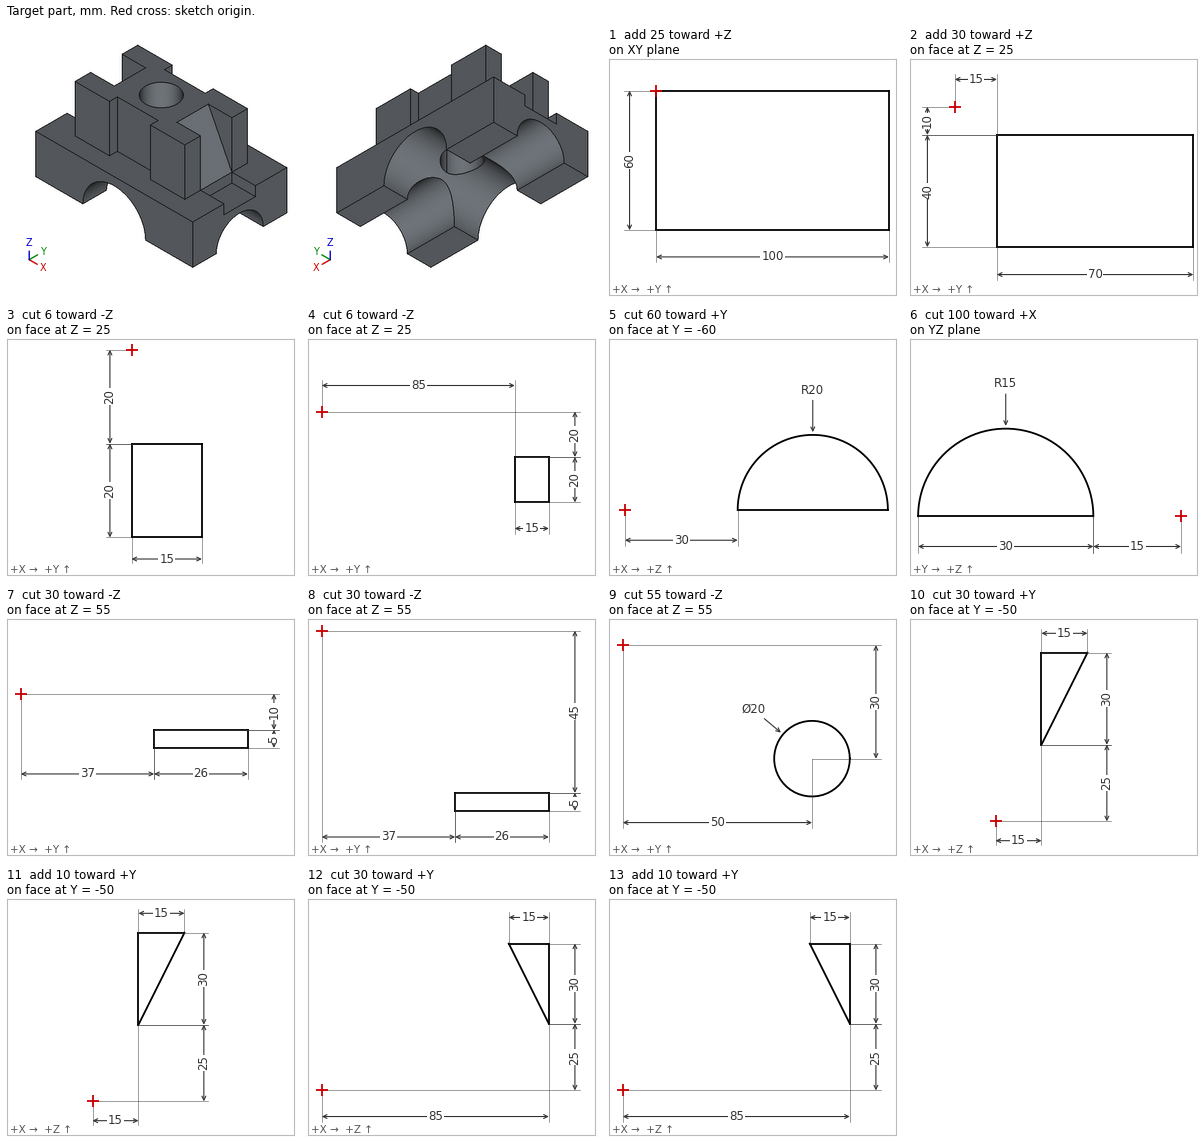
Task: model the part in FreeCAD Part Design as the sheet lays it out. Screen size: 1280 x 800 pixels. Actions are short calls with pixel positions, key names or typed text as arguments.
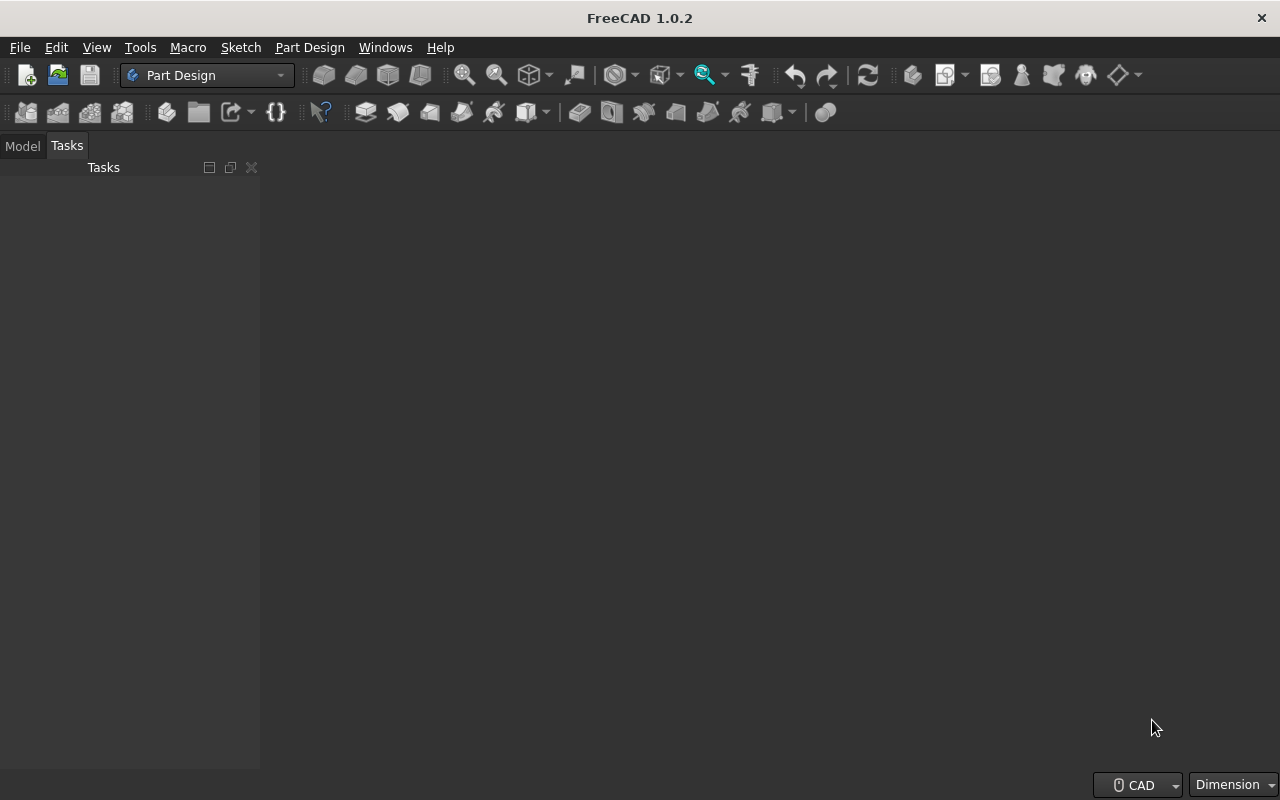
key(ctrl+n)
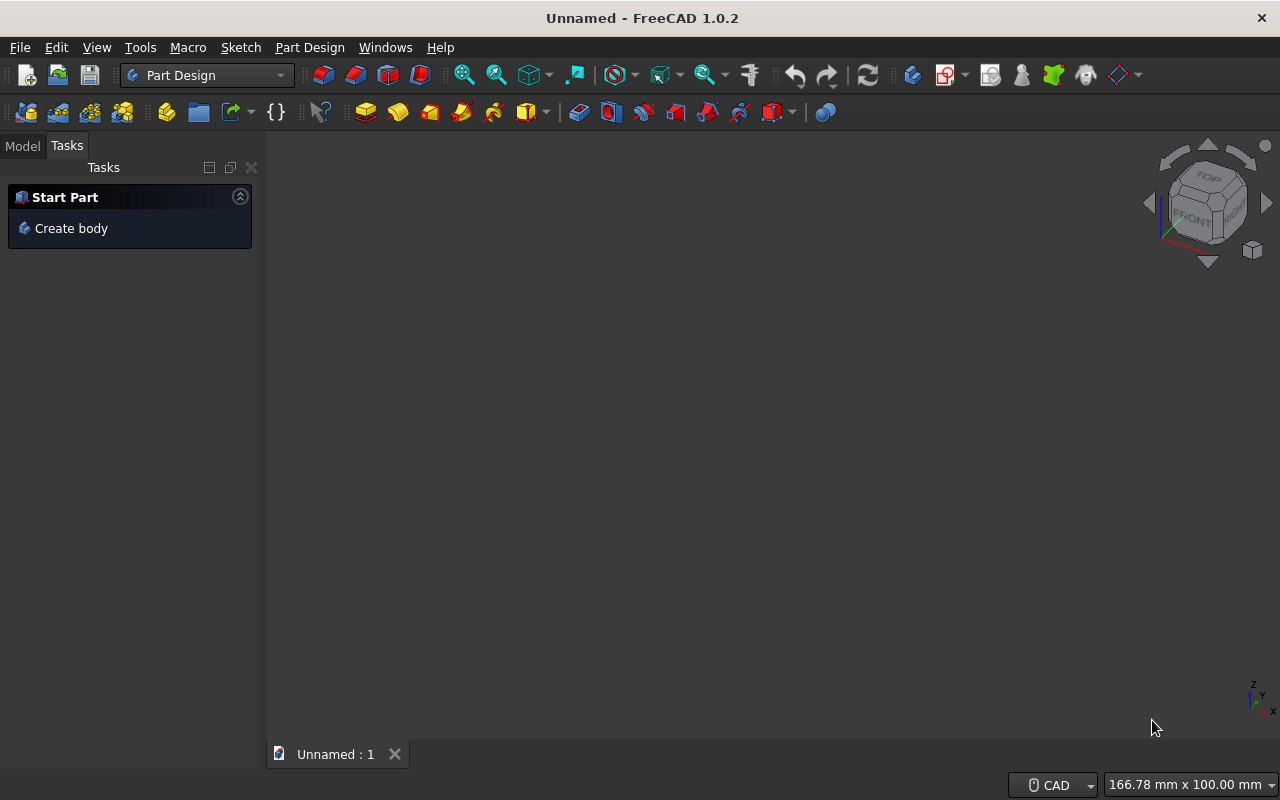
click(946, 76)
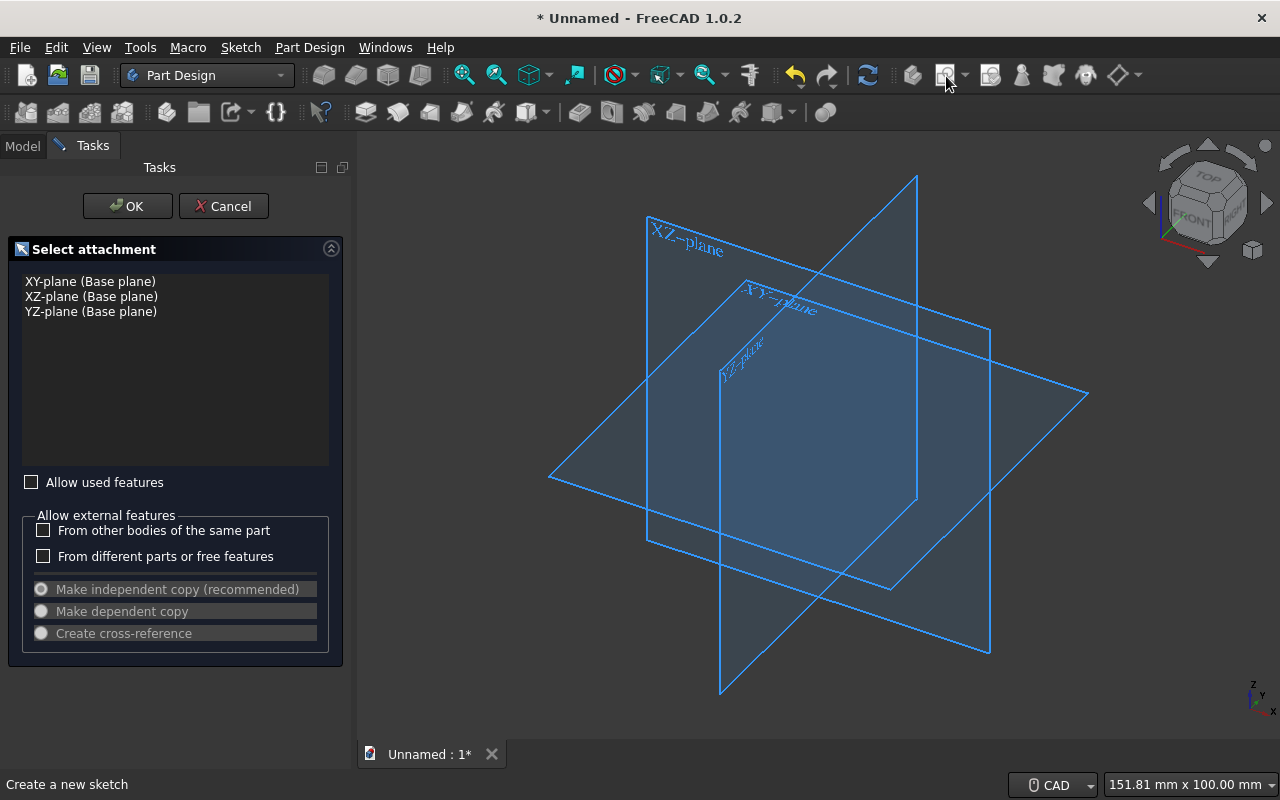
click(82, 282)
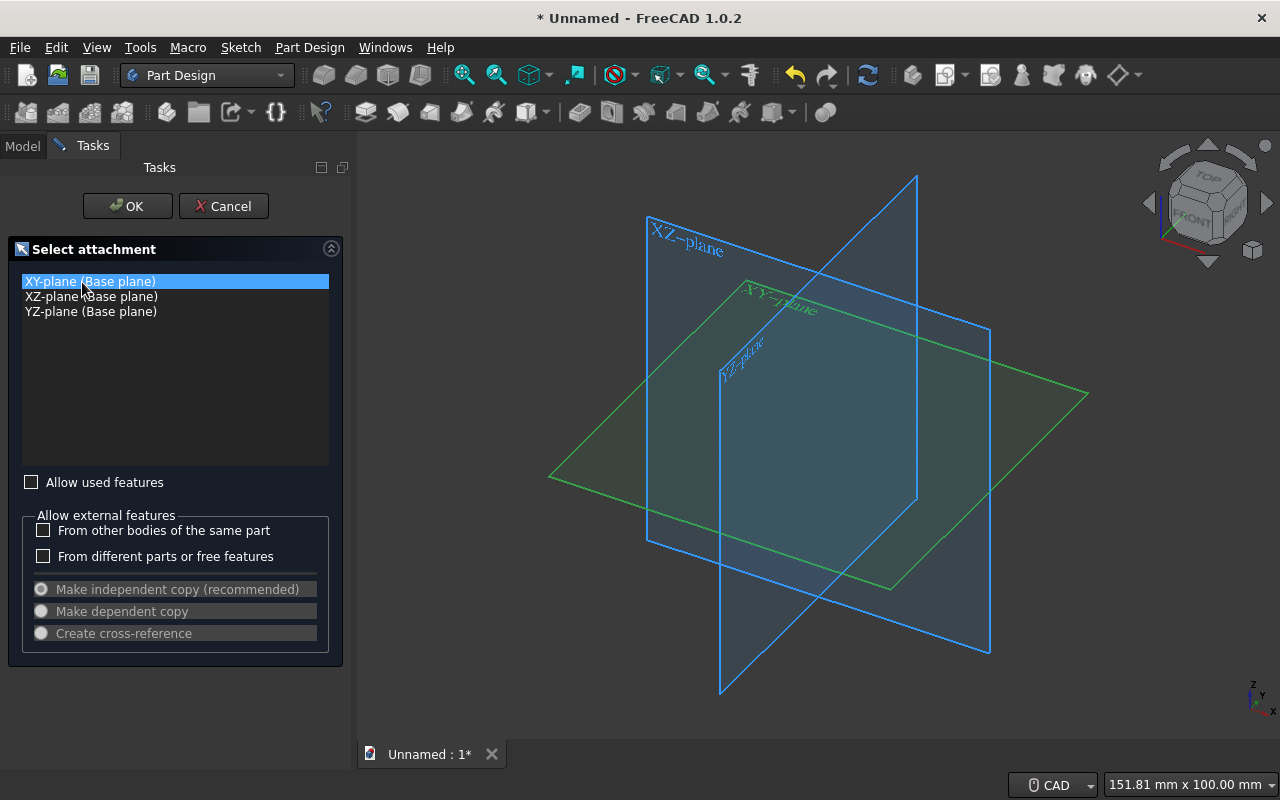
click(128, 206)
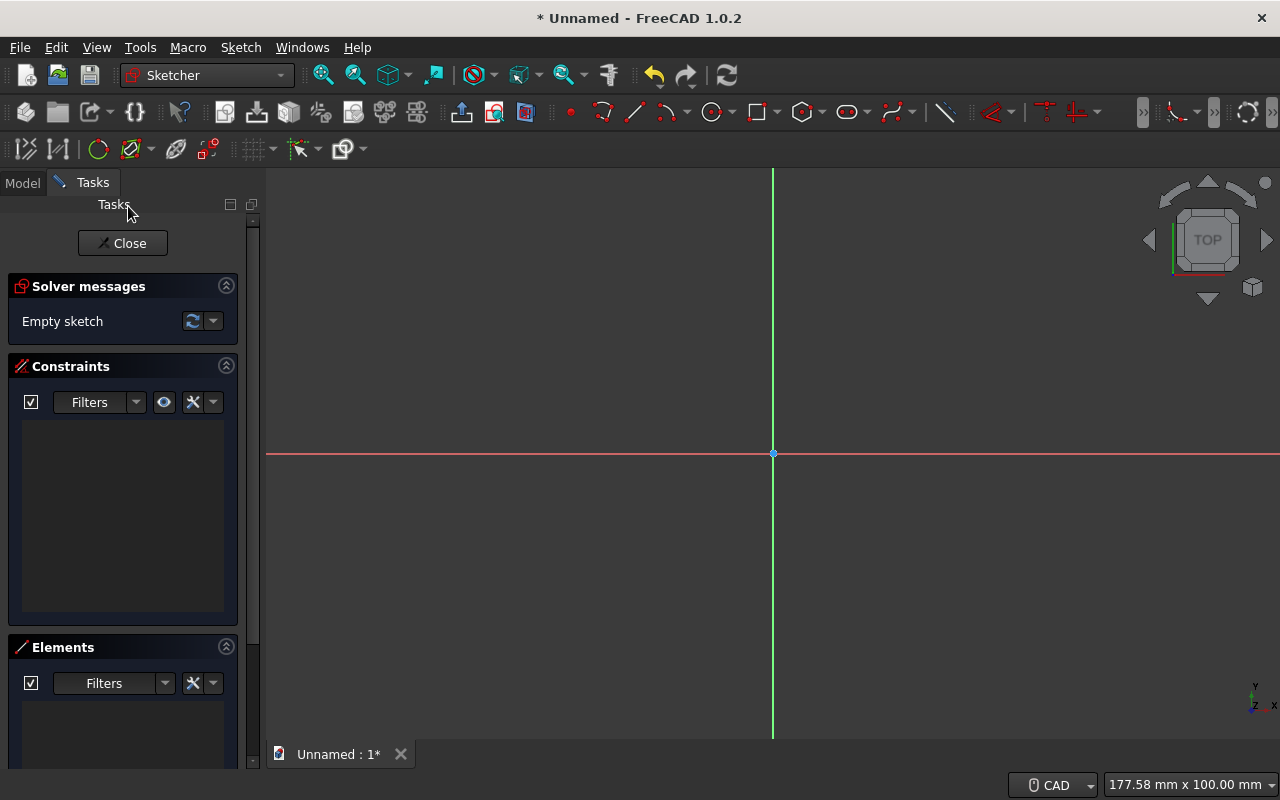
scroll(294, 196, down, 2)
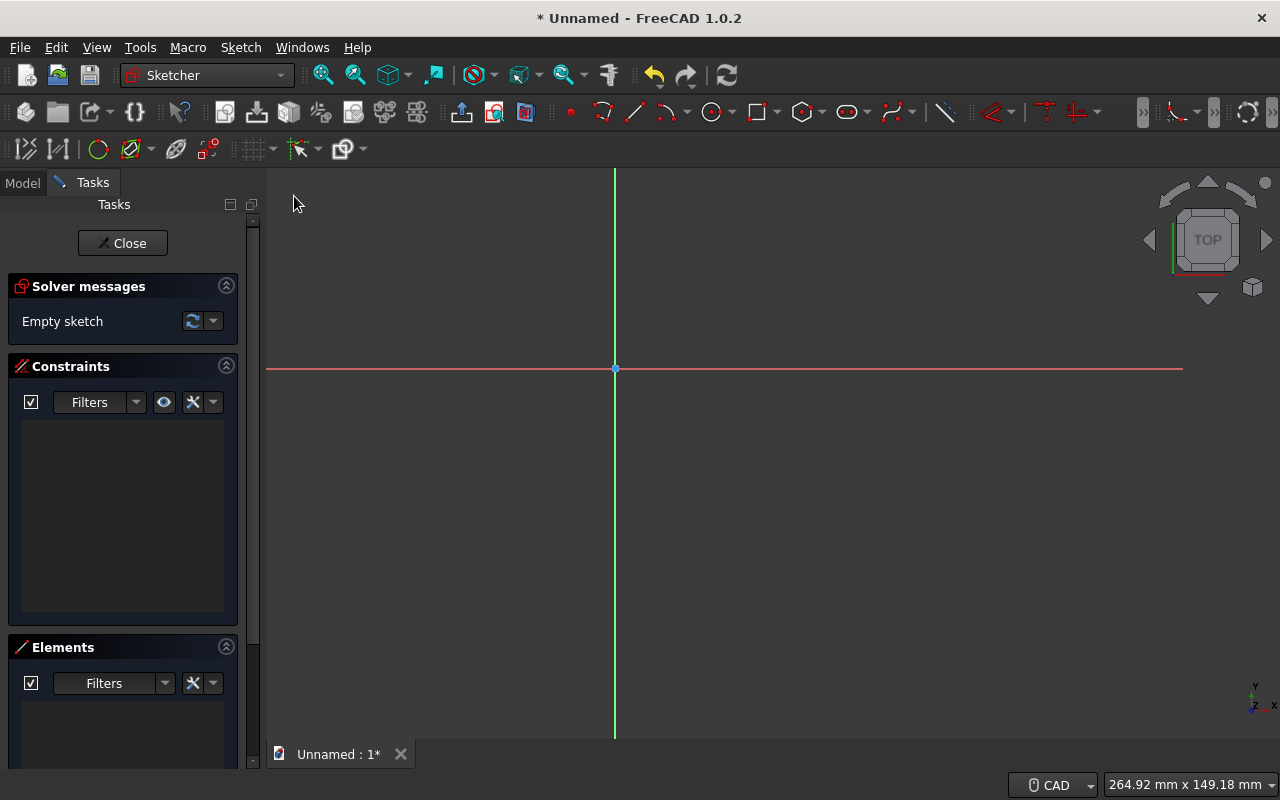
scroll(1014, 544, up, 2)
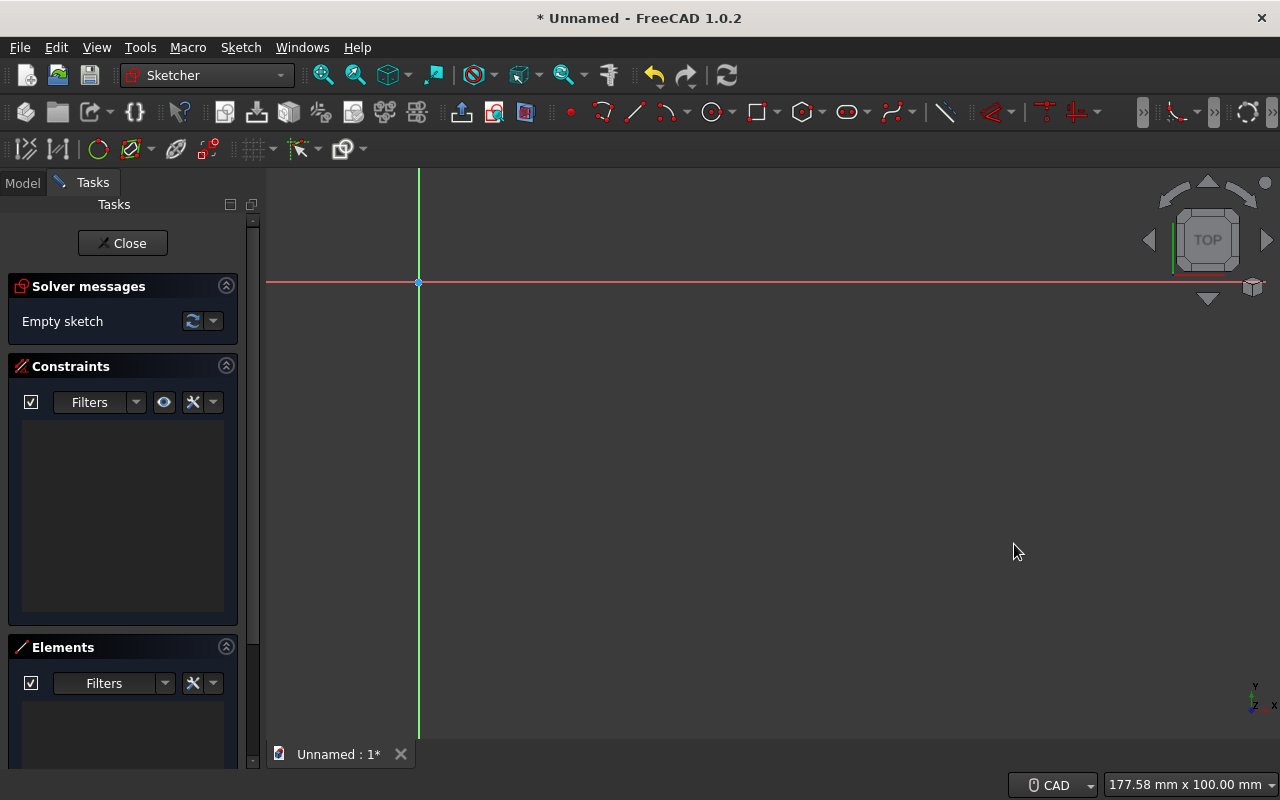
key(g)
key(r)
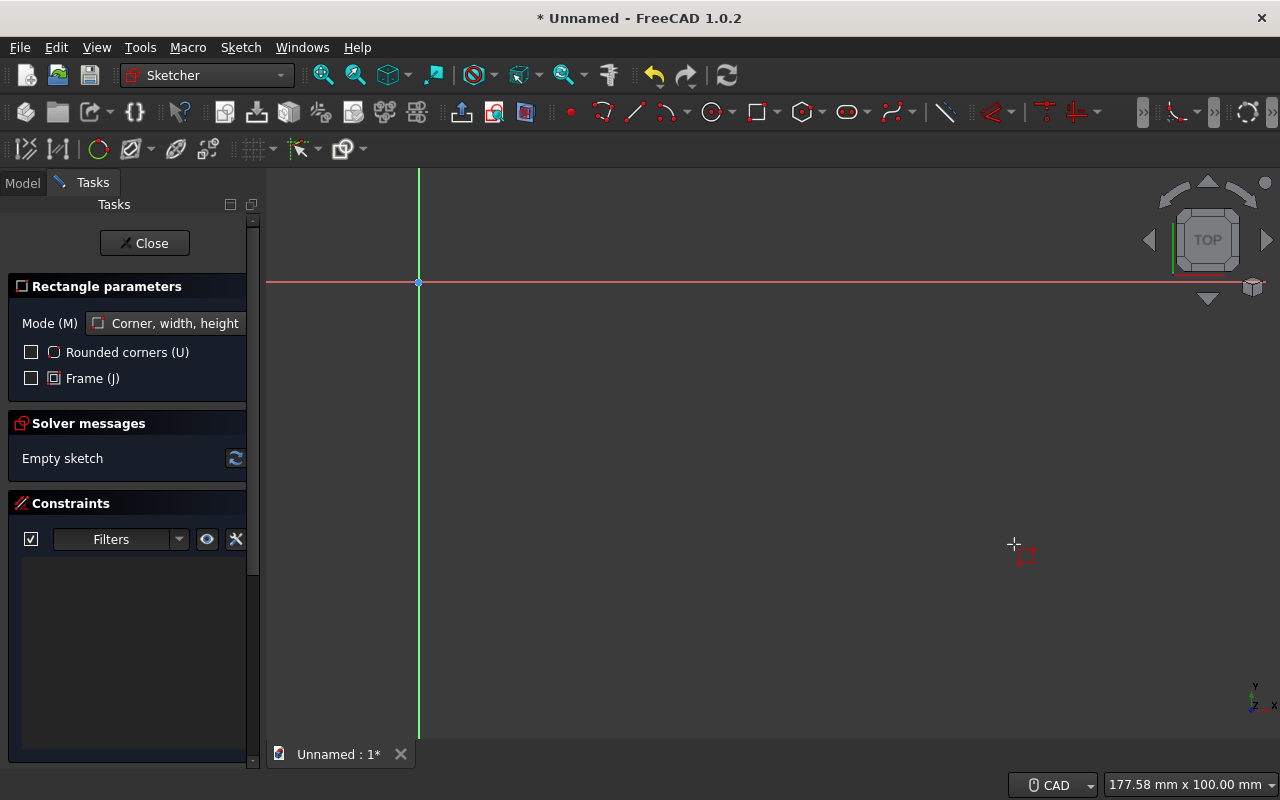
click(419, 282)
click(990, 625)
key(Escape)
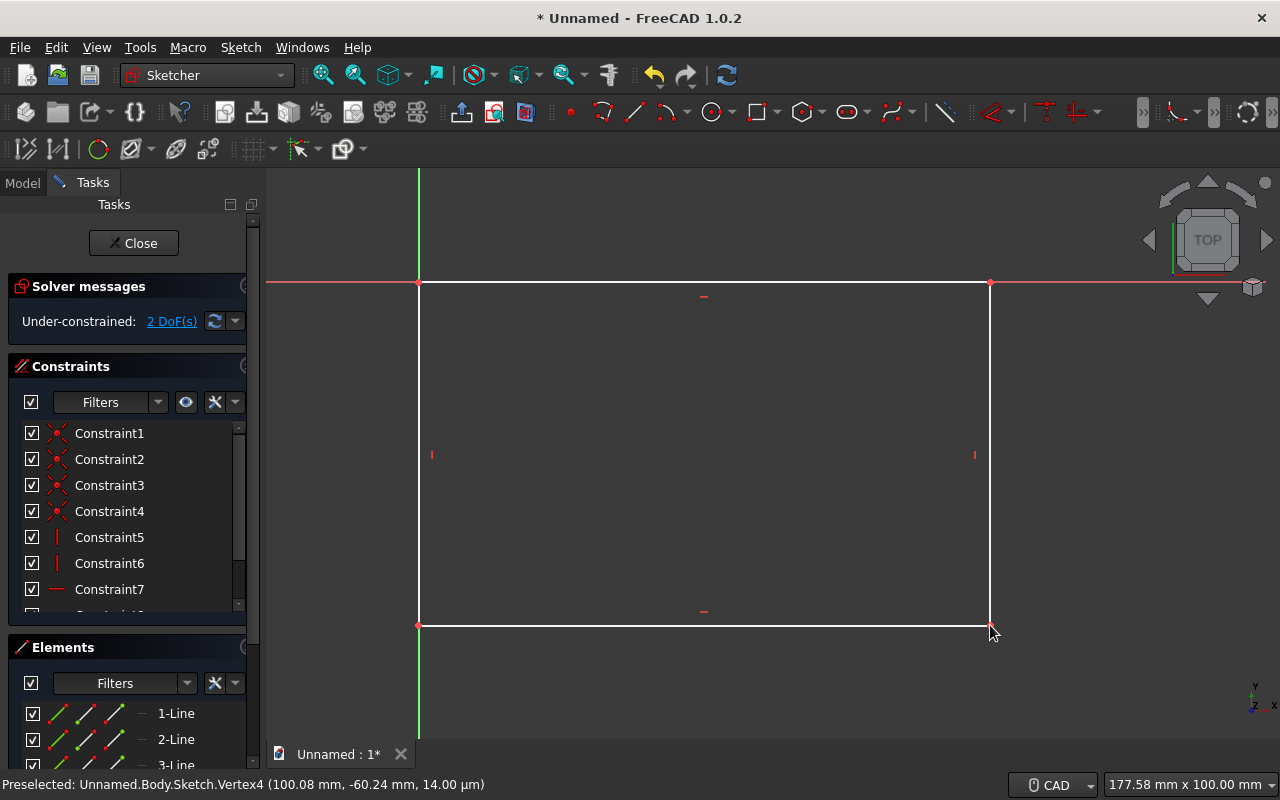
key(d)